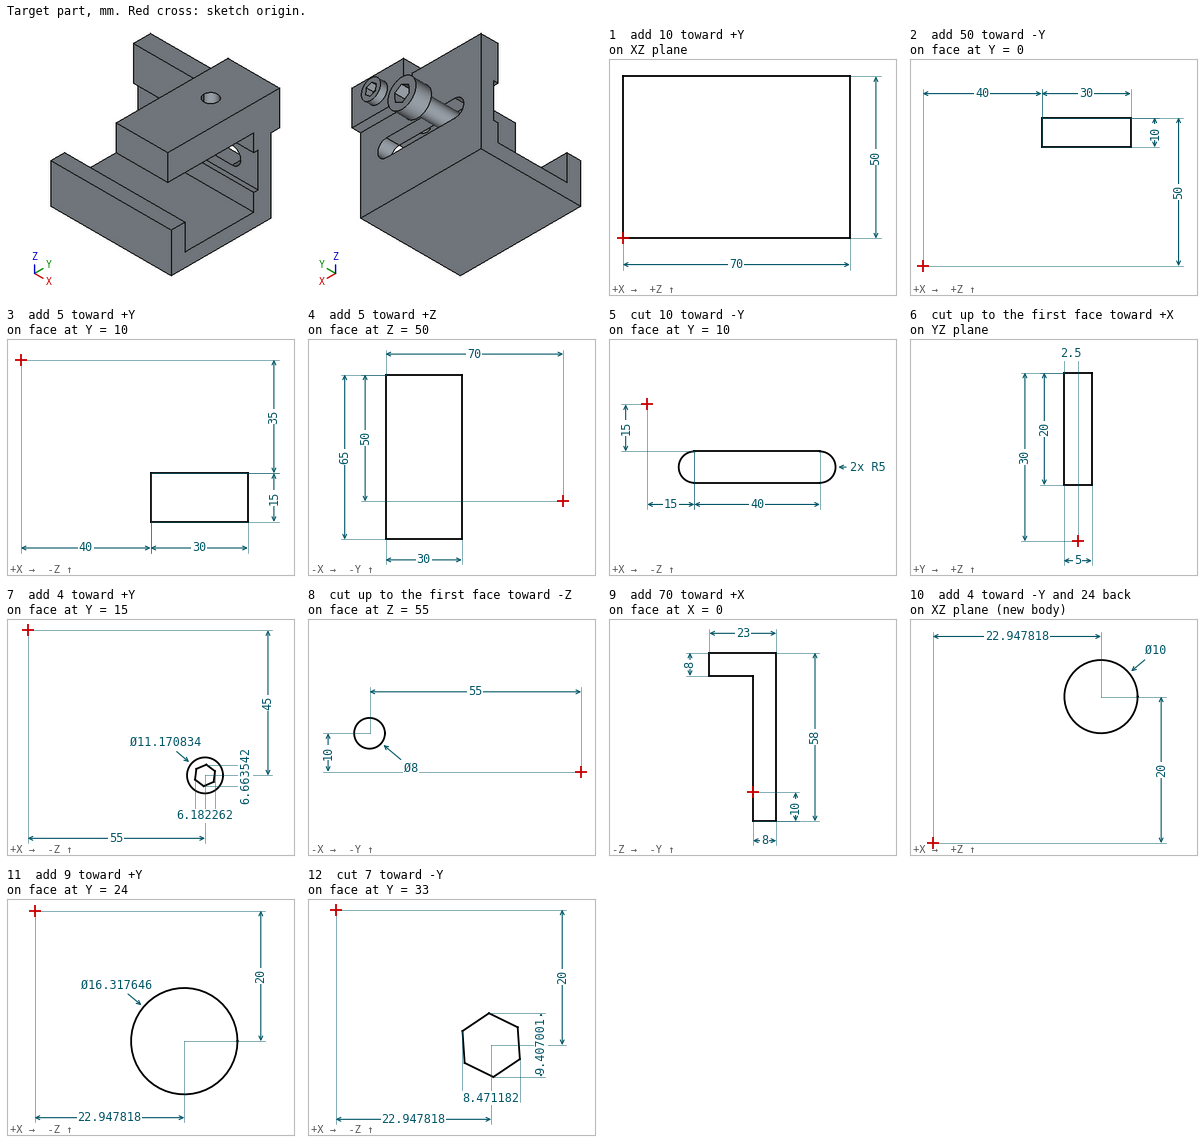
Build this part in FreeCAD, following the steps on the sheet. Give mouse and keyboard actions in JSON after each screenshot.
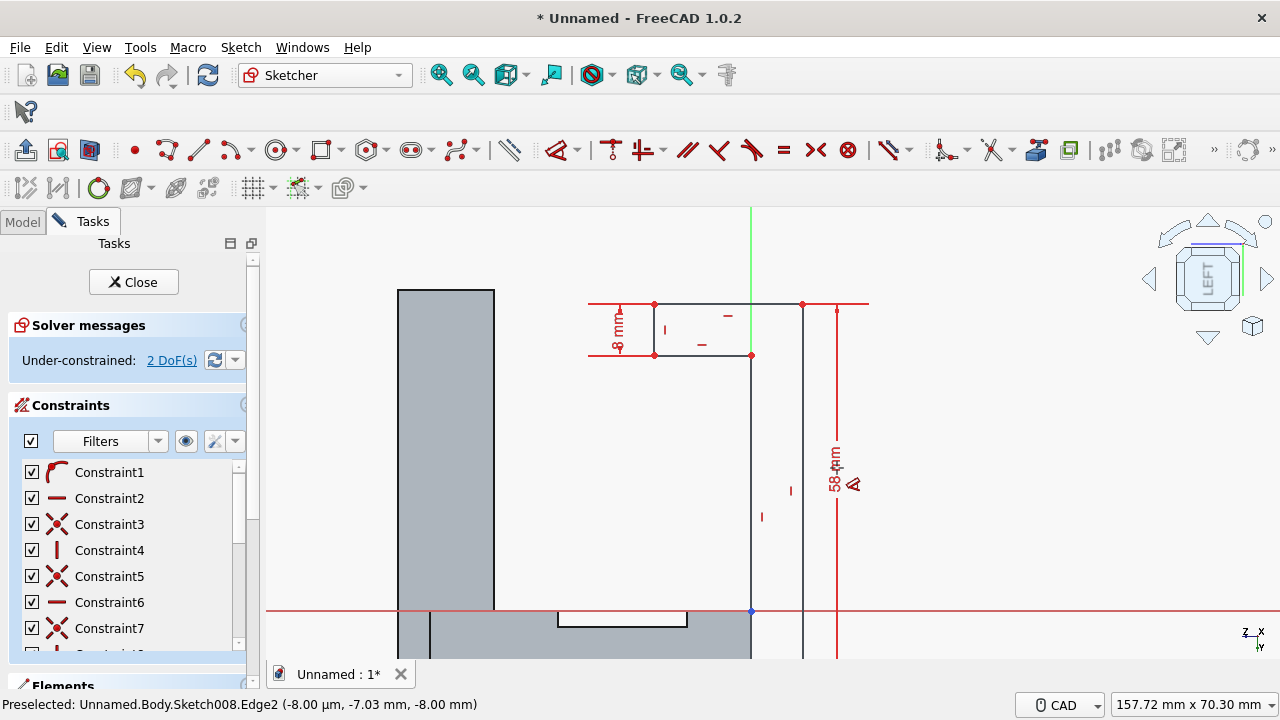
{"action": "left_click", "coordinate": [699, 304]}
{"action": "left_click", "coordinate": [729, 270]}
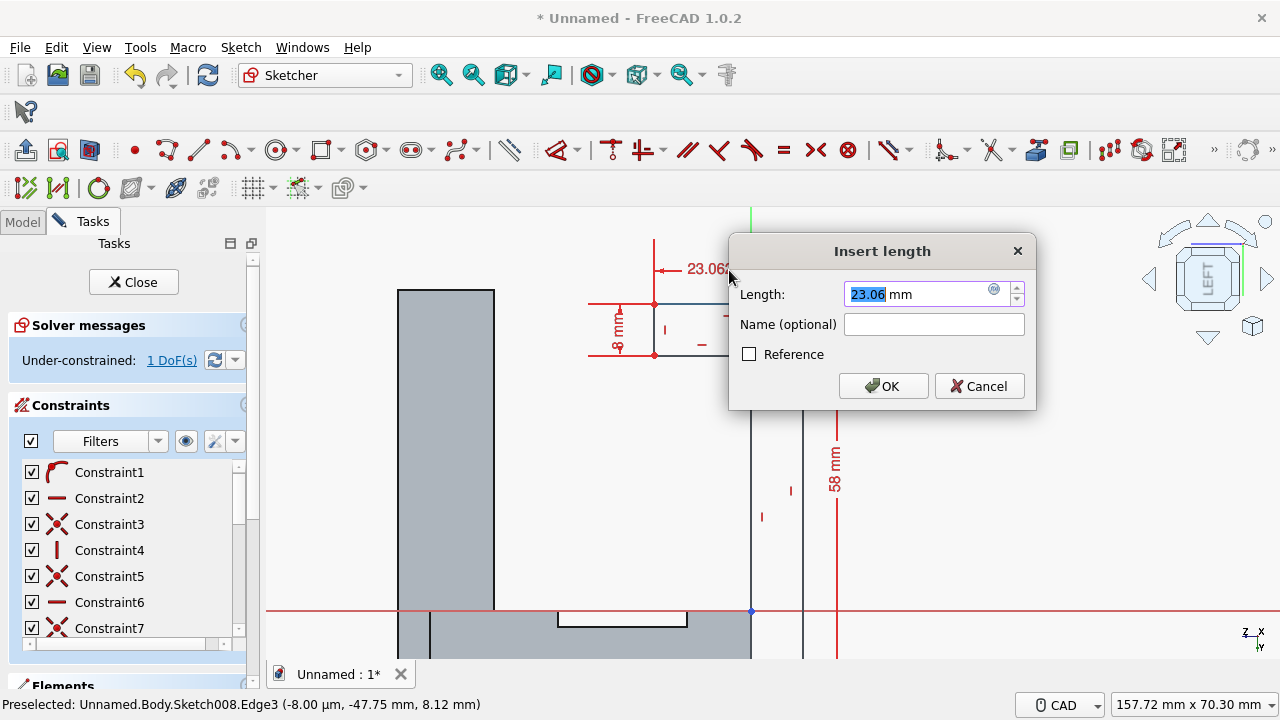
{"action": "type", "text": "23"}
{"action": "key", "text": "Return"}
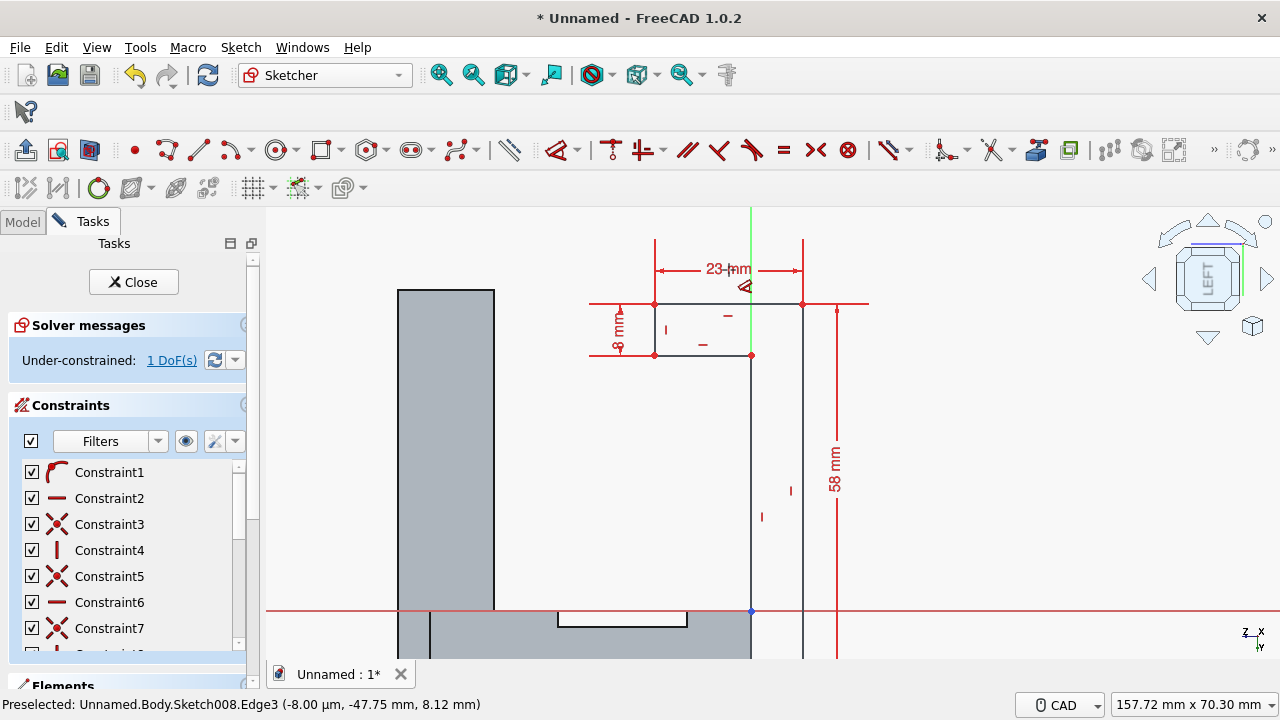
{"action": "scroll", "coordinate": [595, 235], "scroll_direction": "down", "scroll_amount": 1}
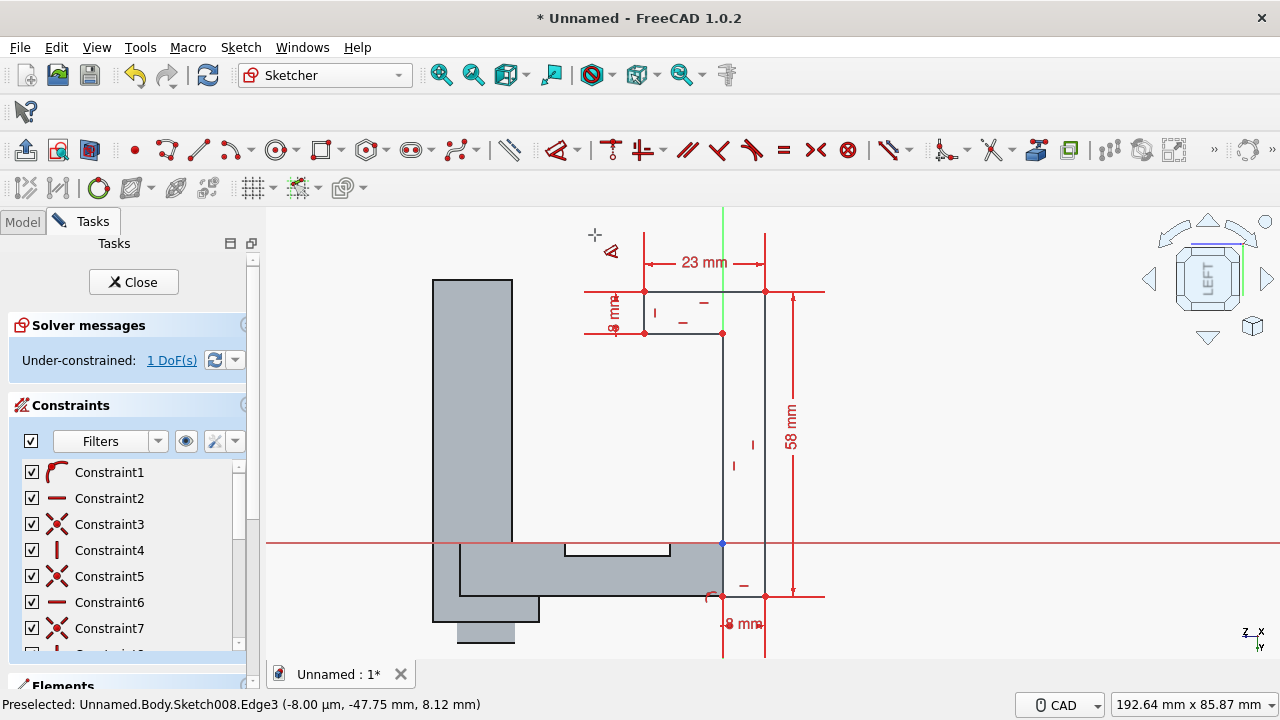
{"action": "left_click", "coordinate": [723, 597]}
{"action": "left_click", "coordinate": [689, 570]}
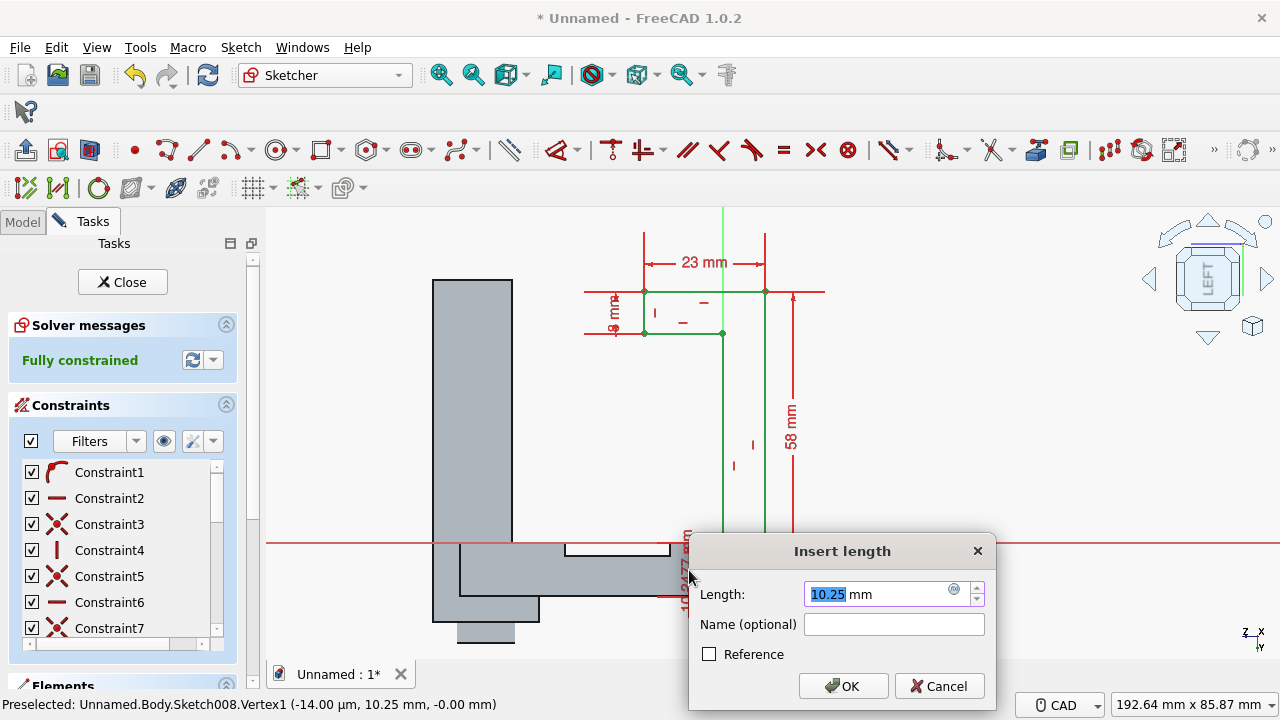
{"action": "type", "text": "10"}
{"action": "key", "text": "Return"}
{"action": "key", "text": "Escape"}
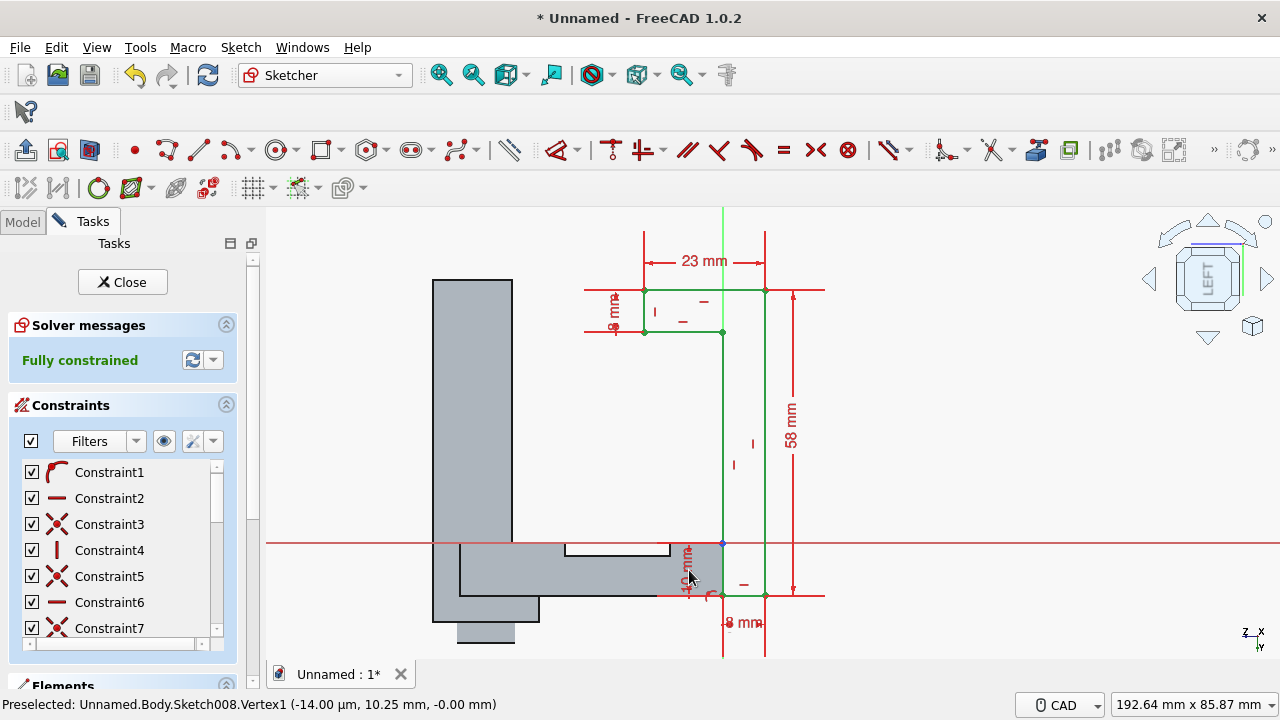
{"action": "left_click", "coordinate": [123, 282]}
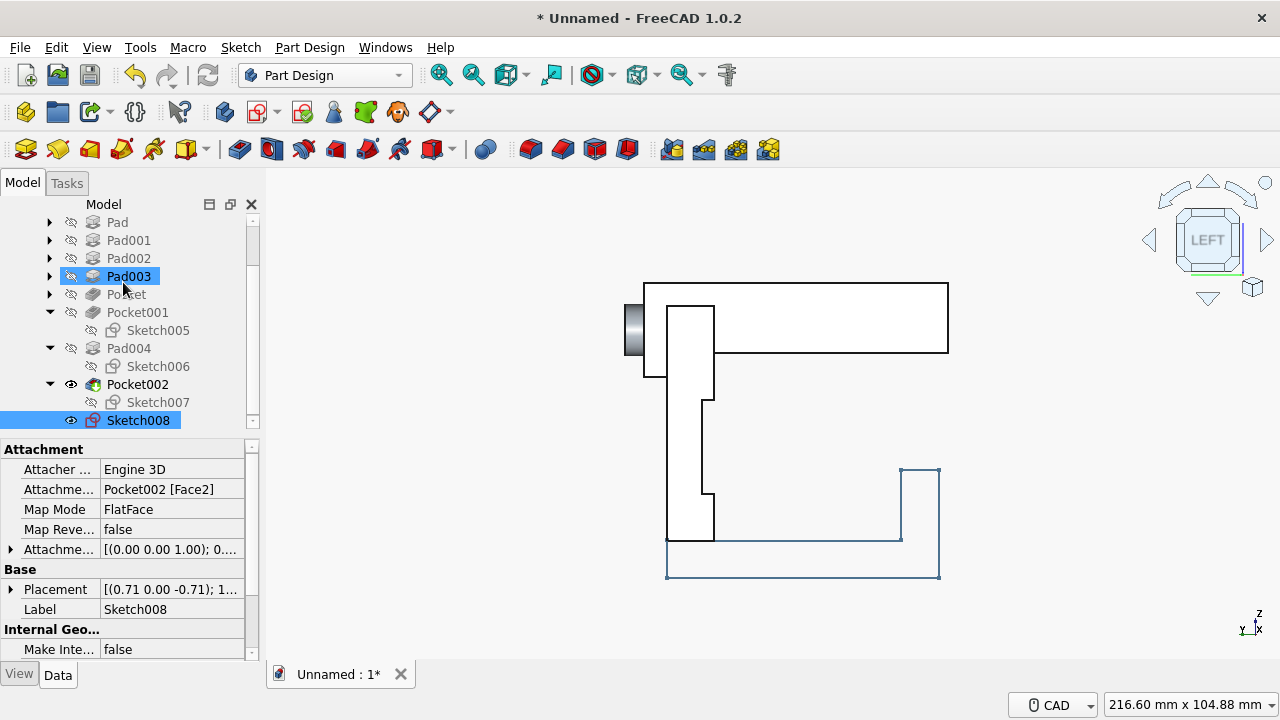
{"action": "left_click", "coordinate": [26, 150]}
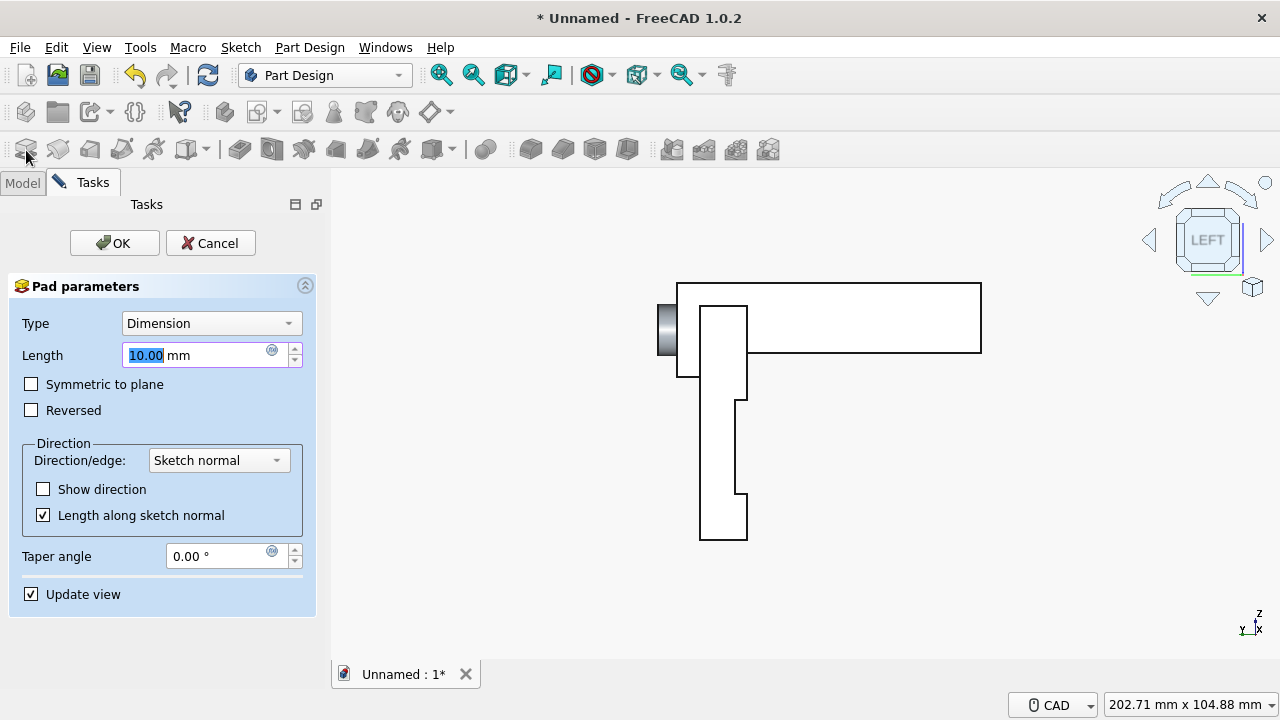
{"action": "type", "text": "70"}
{"action": "key", "text": "Tab"}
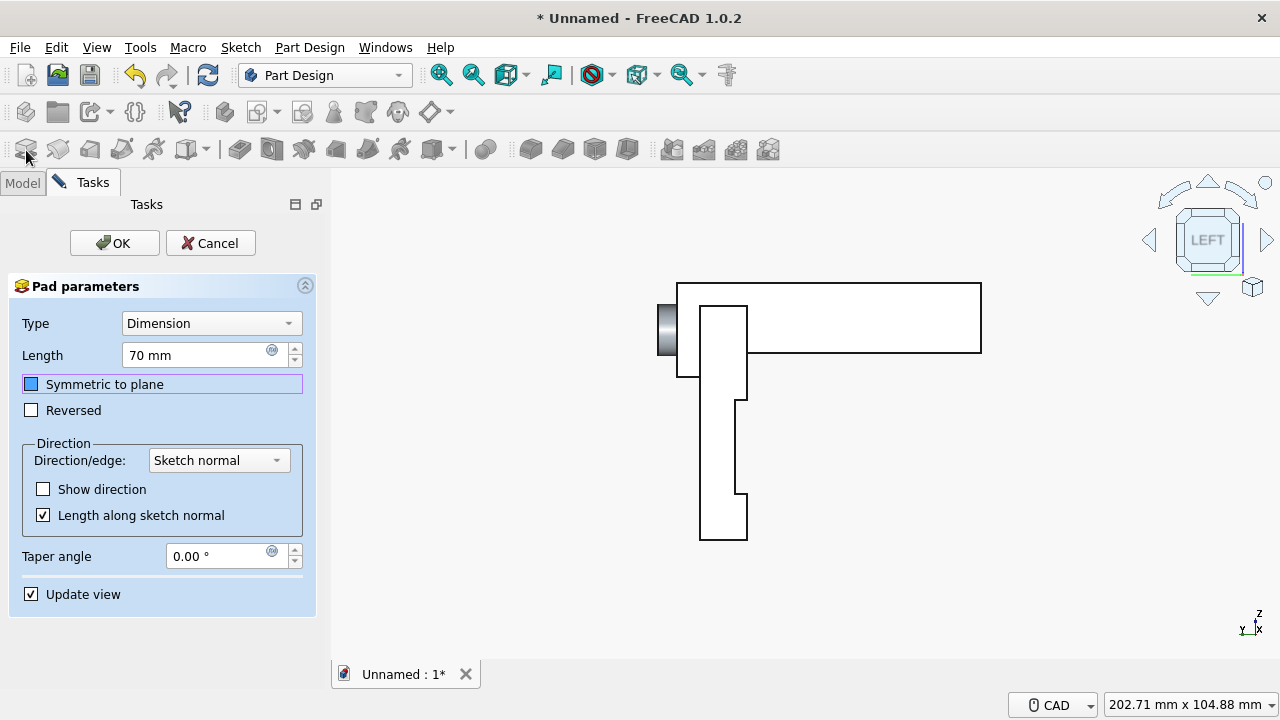
{"action": "left_click", "coordinate": [30, 410]}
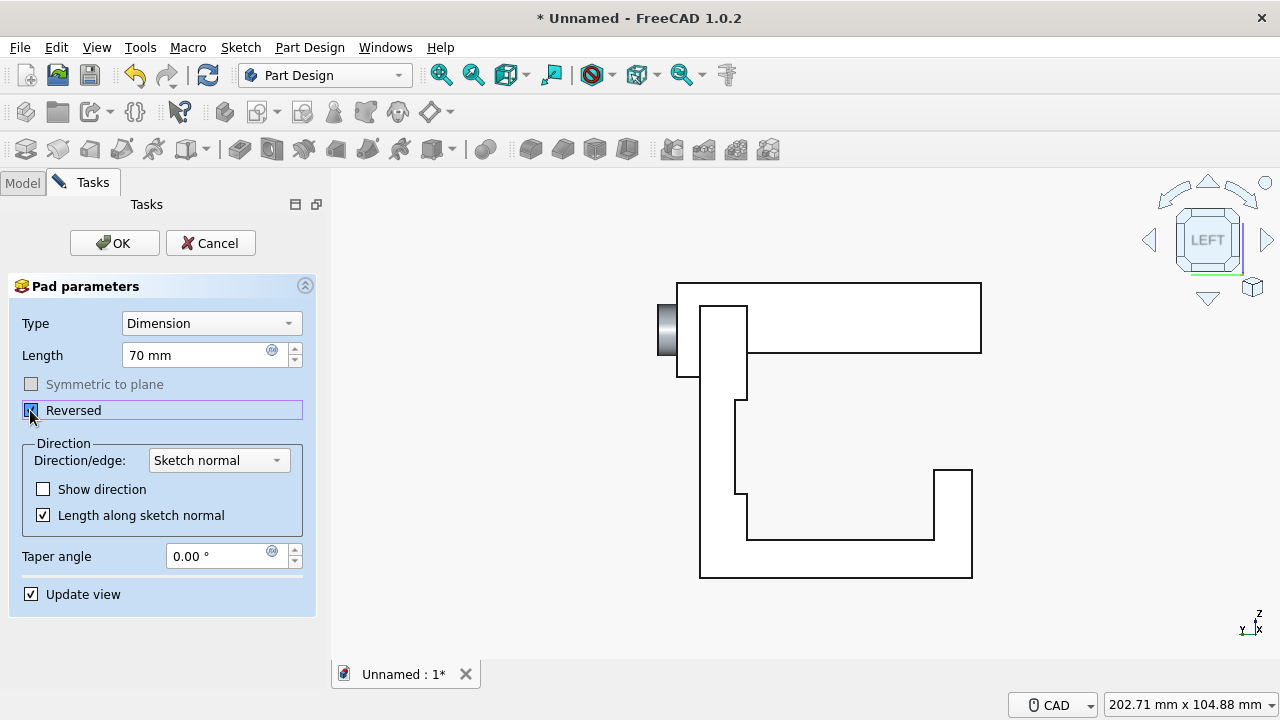
{"action": "left_click", "coordinate": [115, 243]}